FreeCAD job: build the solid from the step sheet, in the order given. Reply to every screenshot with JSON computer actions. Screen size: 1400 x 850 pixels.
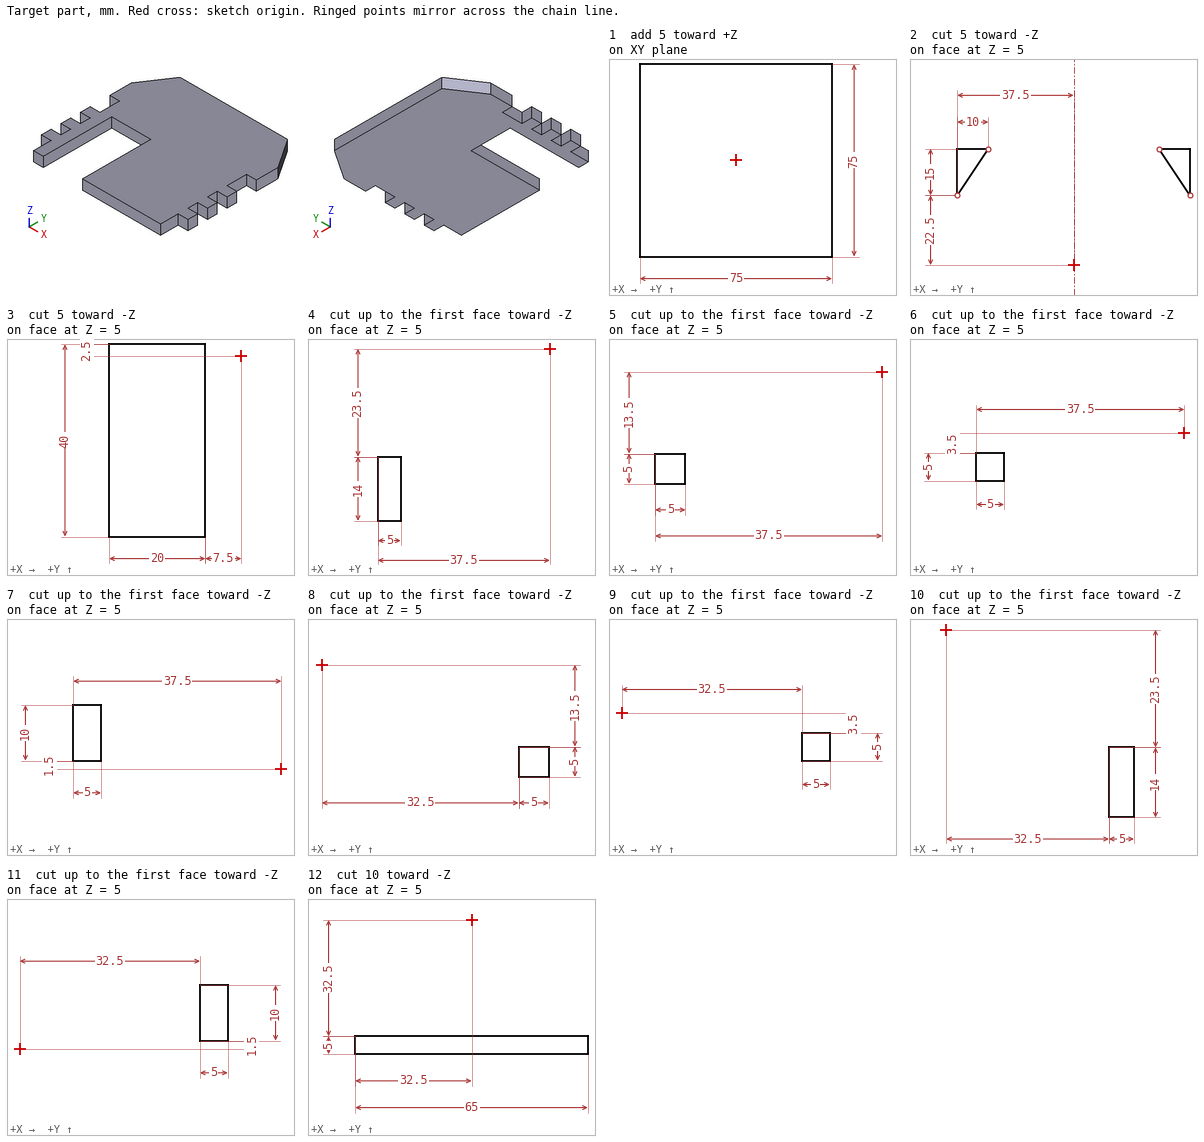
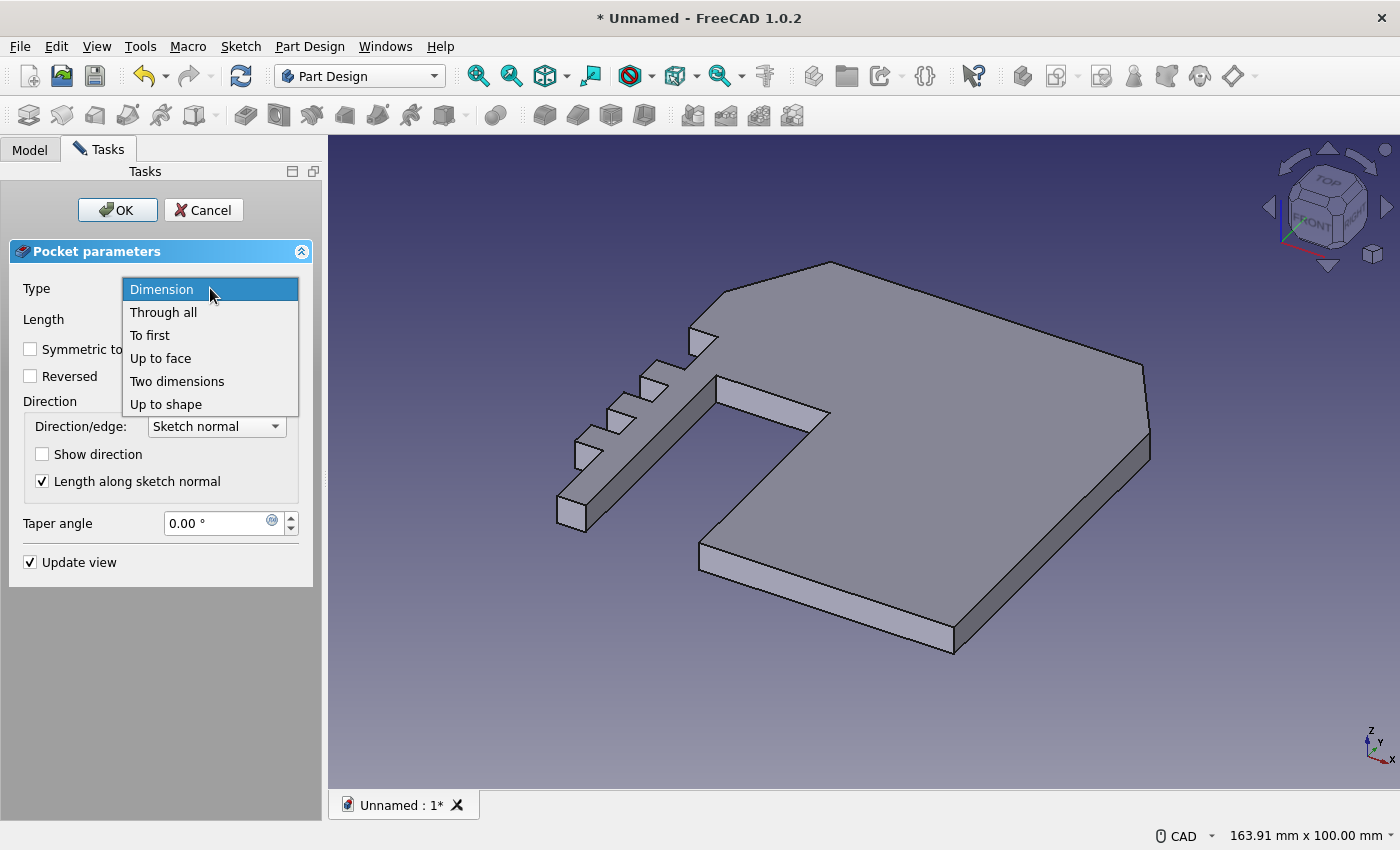
{"action": "left_click", "coordinate": [208, 336]}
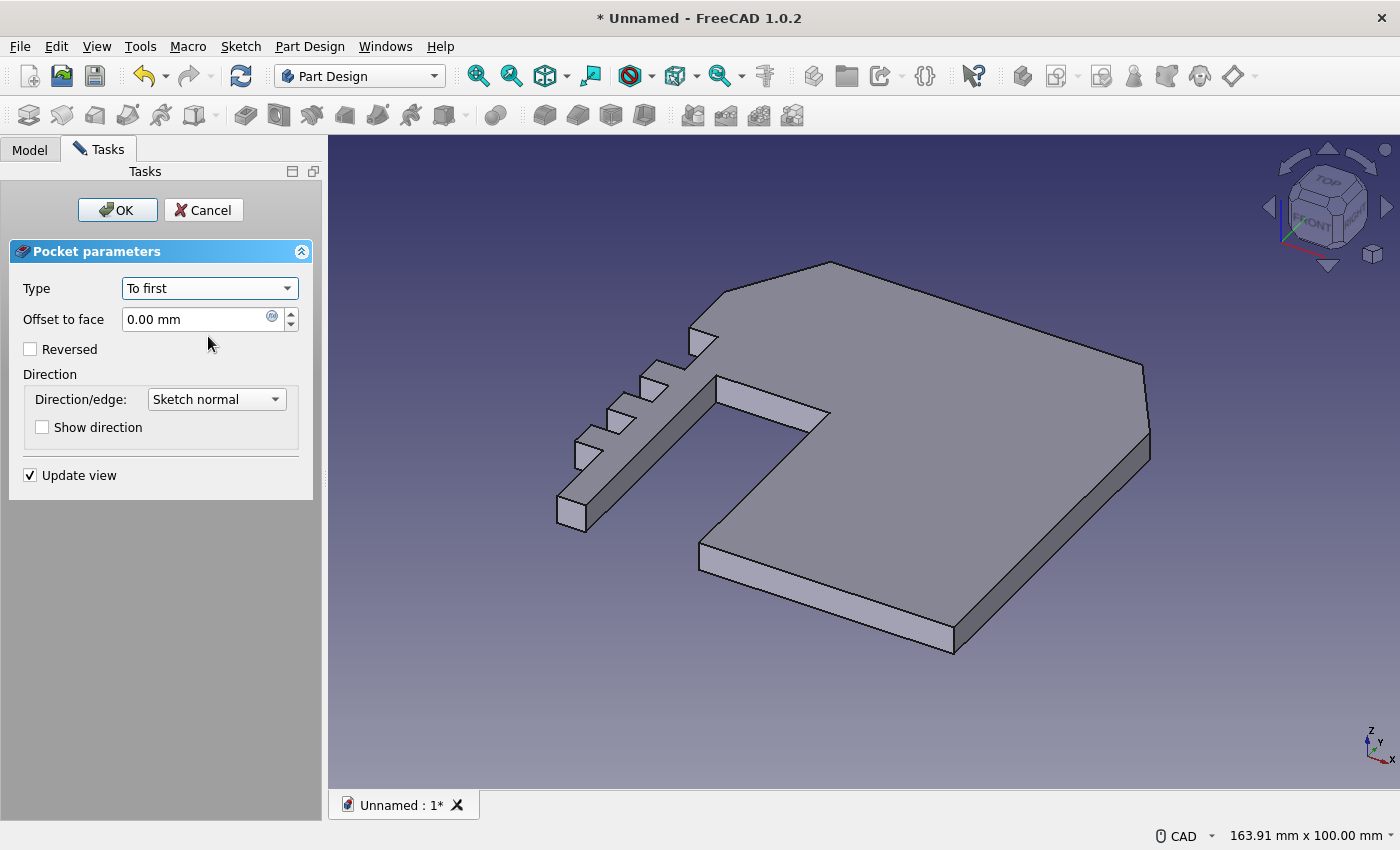
{"action": "left_click", "coordinate": [118, 210]}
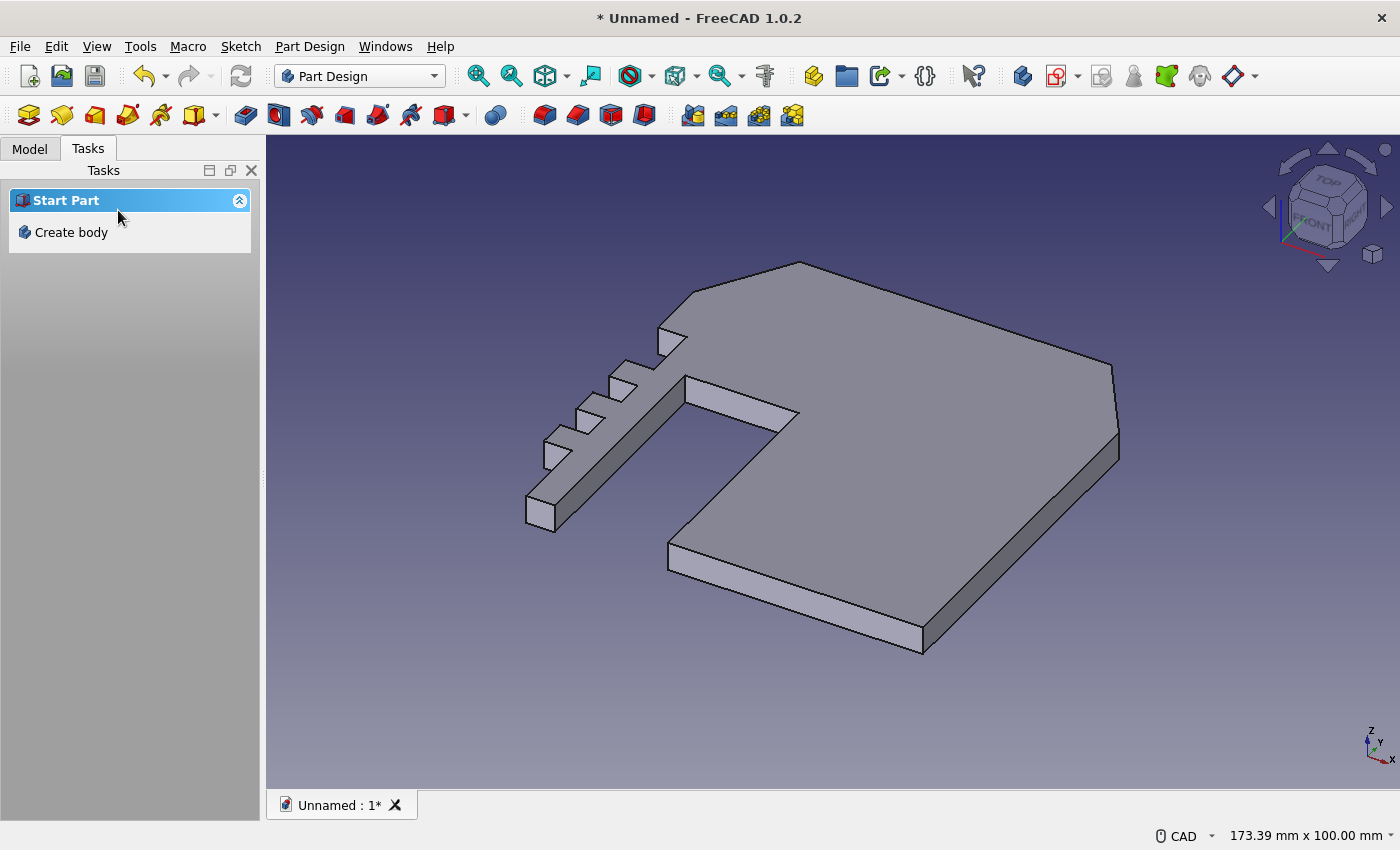
{"action": "left_click", "coordinate": [929, 420]}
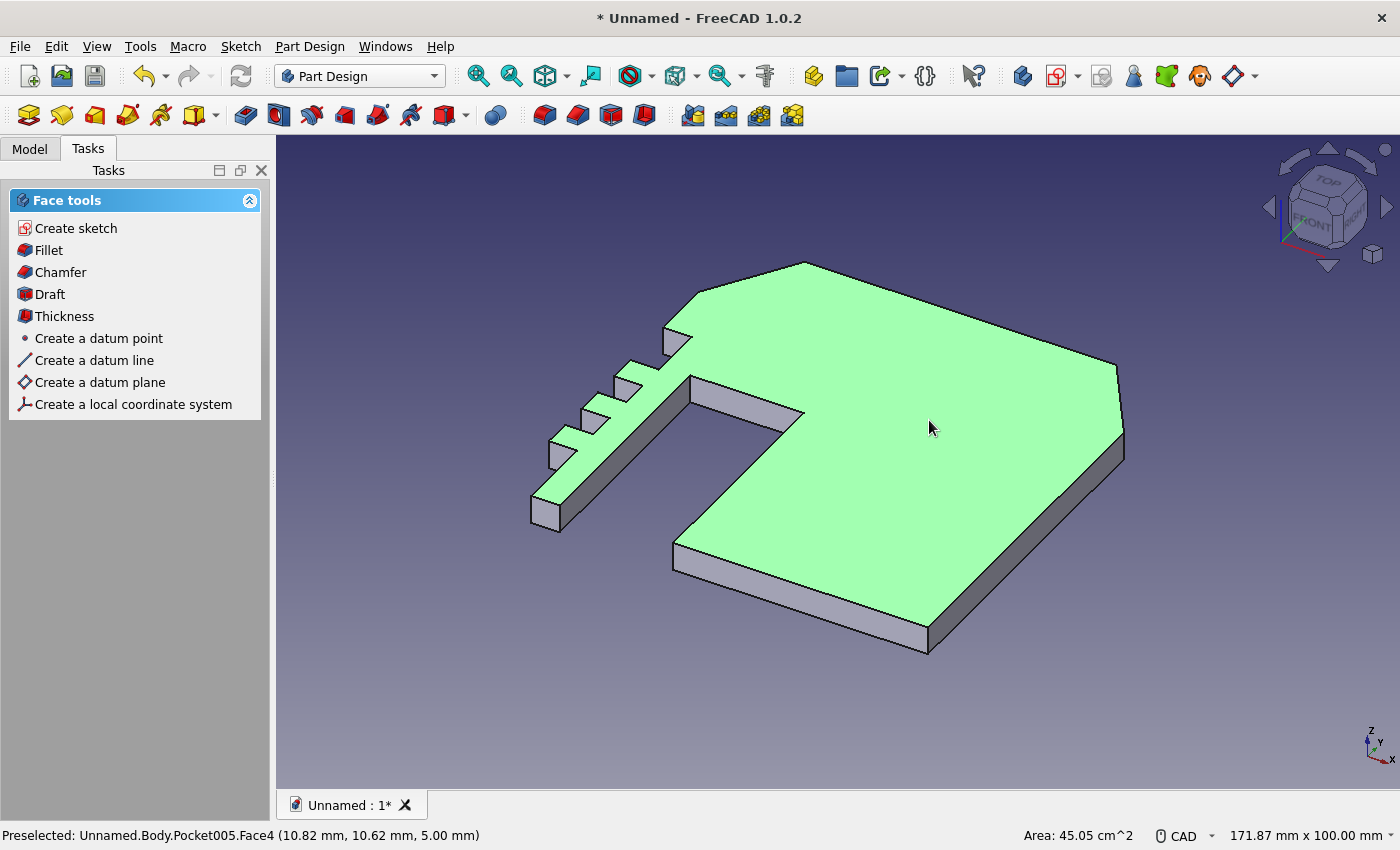
{"action": "left_click", "coordinate": [1056, 76]}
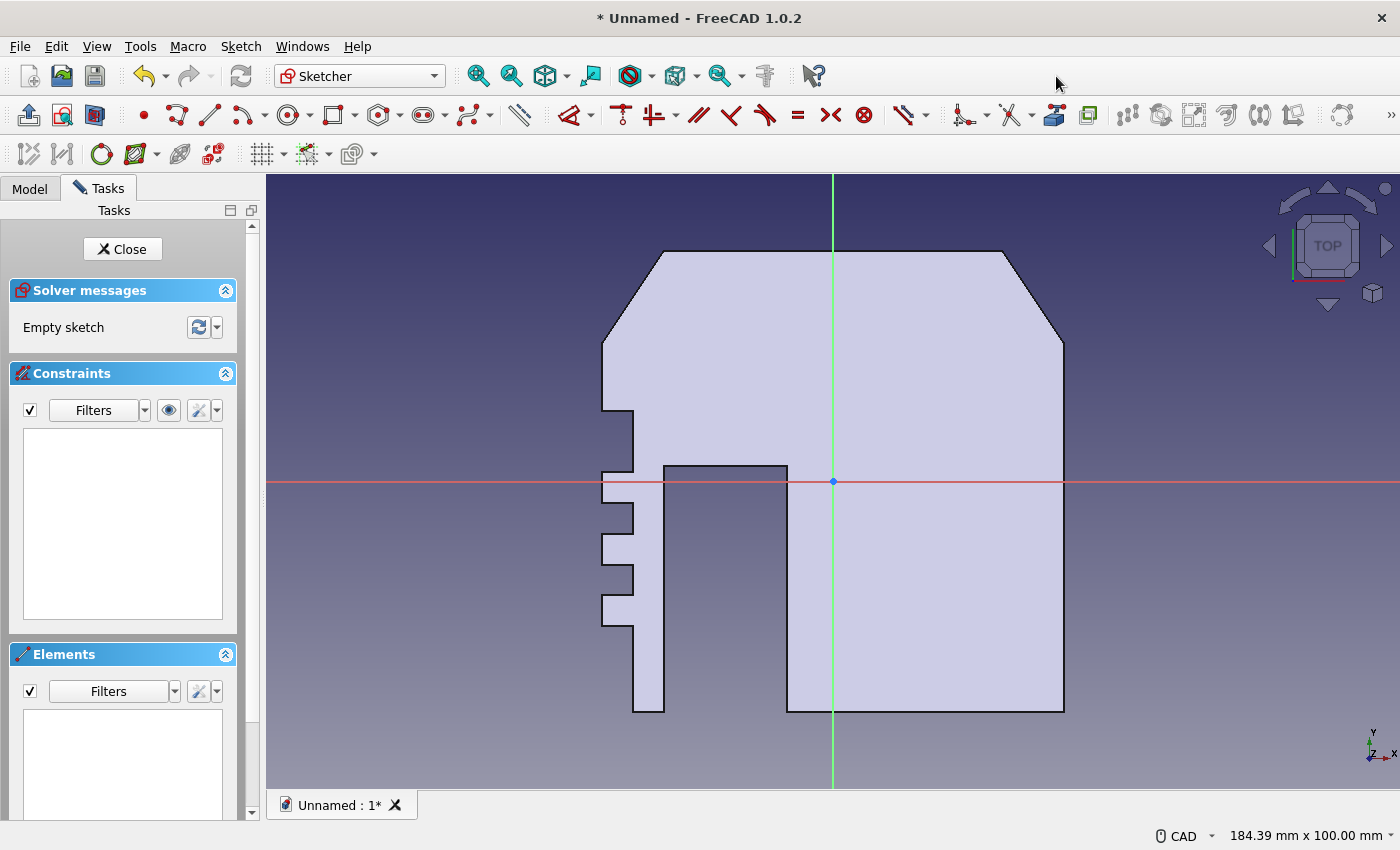
{"action": "scroll", "coordinate": [1071, 588], "scroll_direction": "up", "scroll_amount": 13}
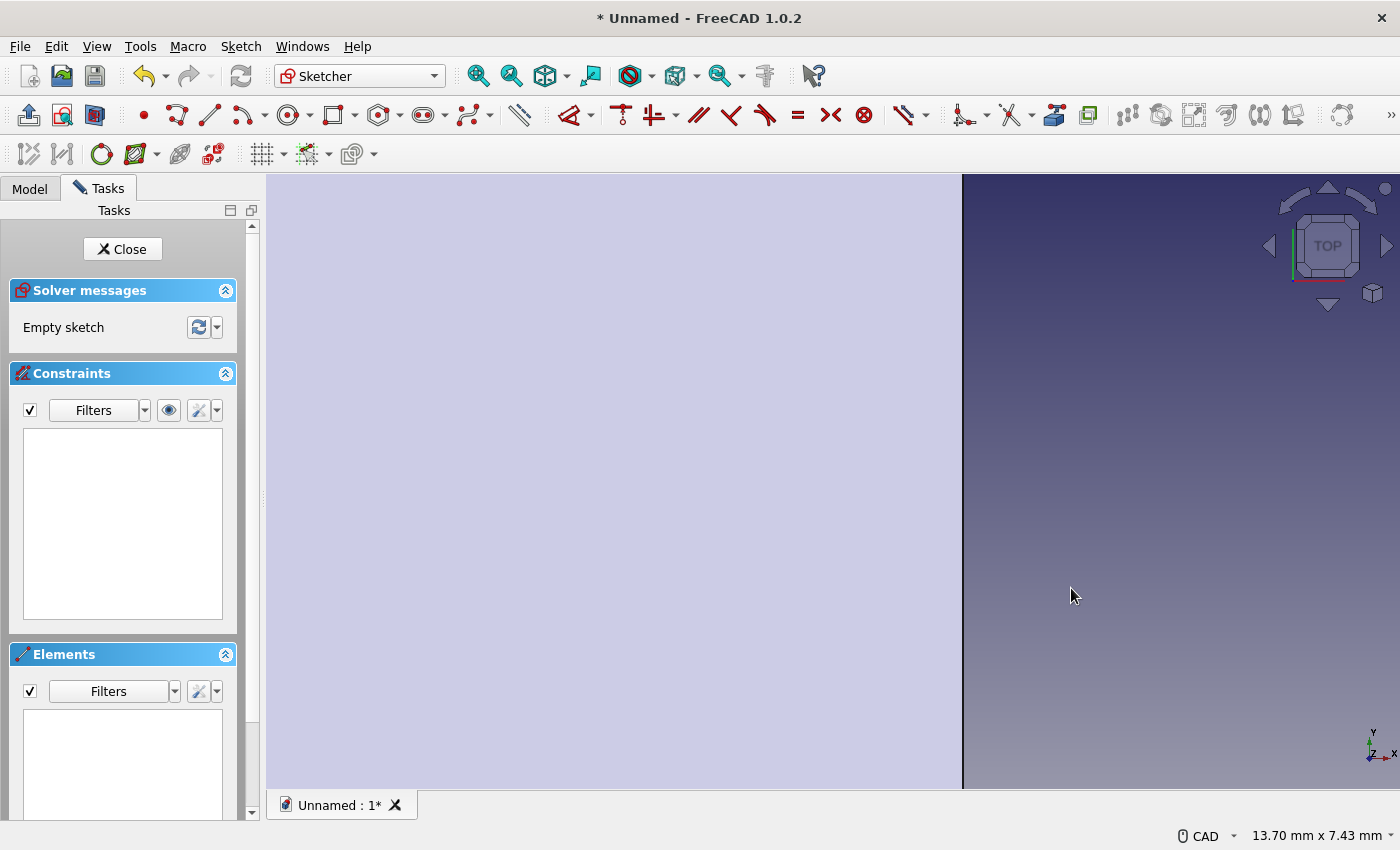
{"action": "left_click", "coordinate": [332, 116]}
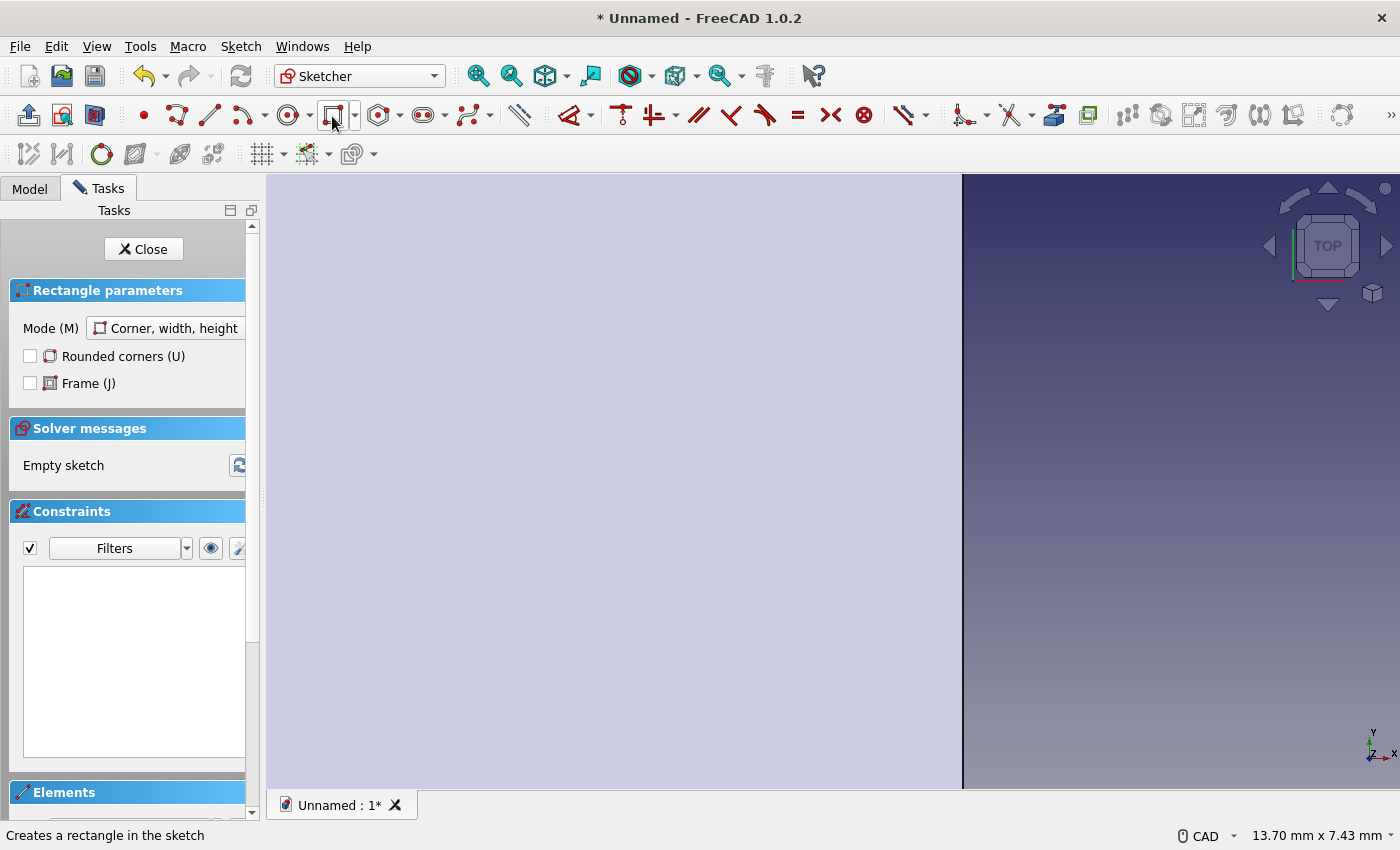
{"action": "left_click", "coordinate": [549, 264]}
{"action": "left_click", "coordinate": [963, 678]}
{"action": "key", "text": "Escape"}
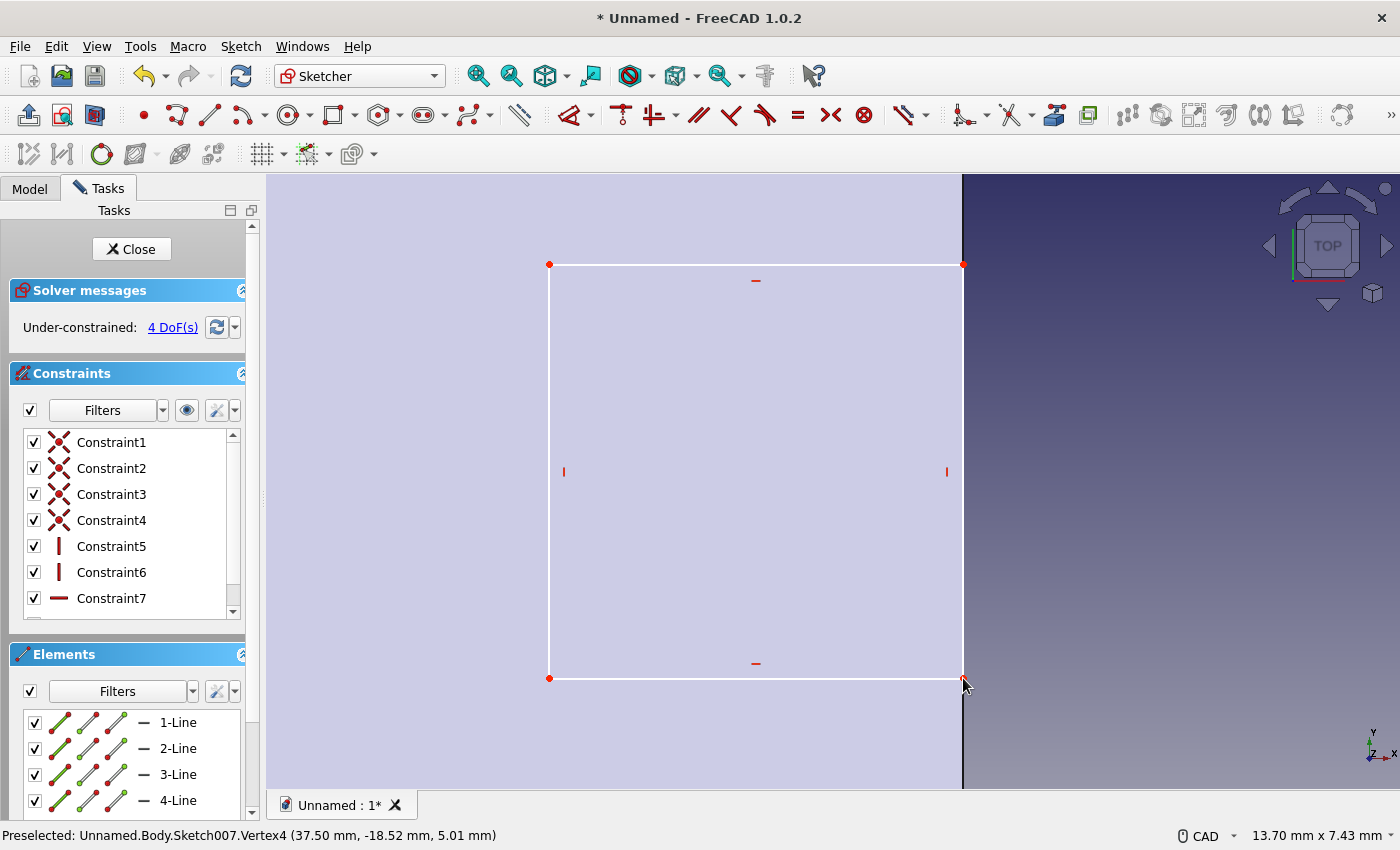
{"action": "left_click", "coordinate": [568, 116]}